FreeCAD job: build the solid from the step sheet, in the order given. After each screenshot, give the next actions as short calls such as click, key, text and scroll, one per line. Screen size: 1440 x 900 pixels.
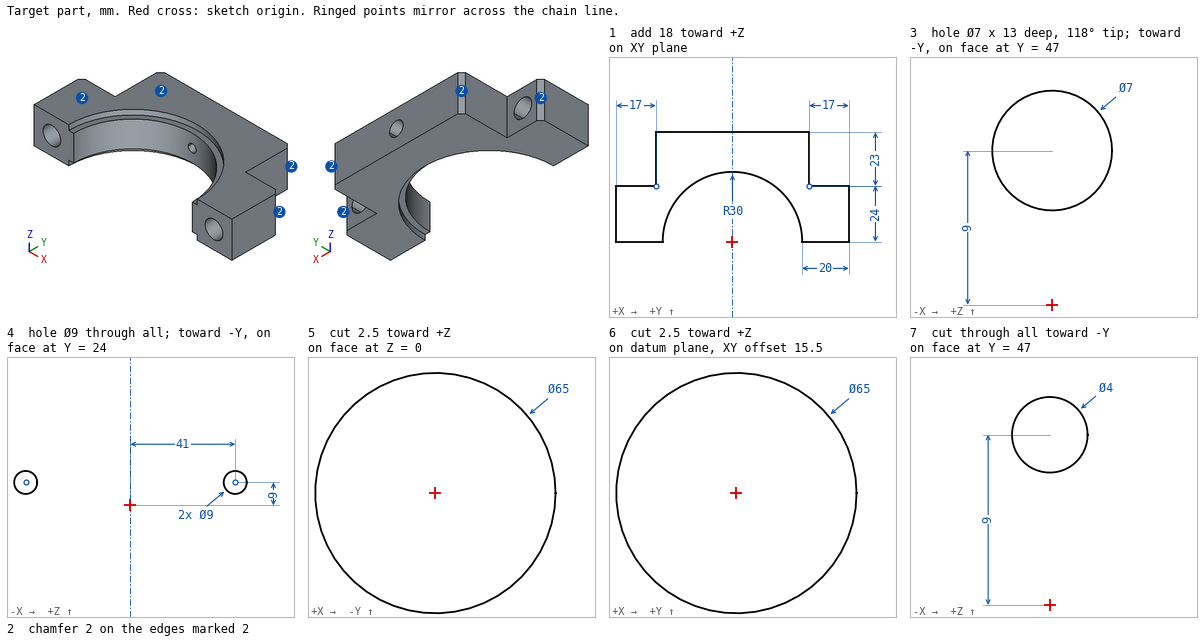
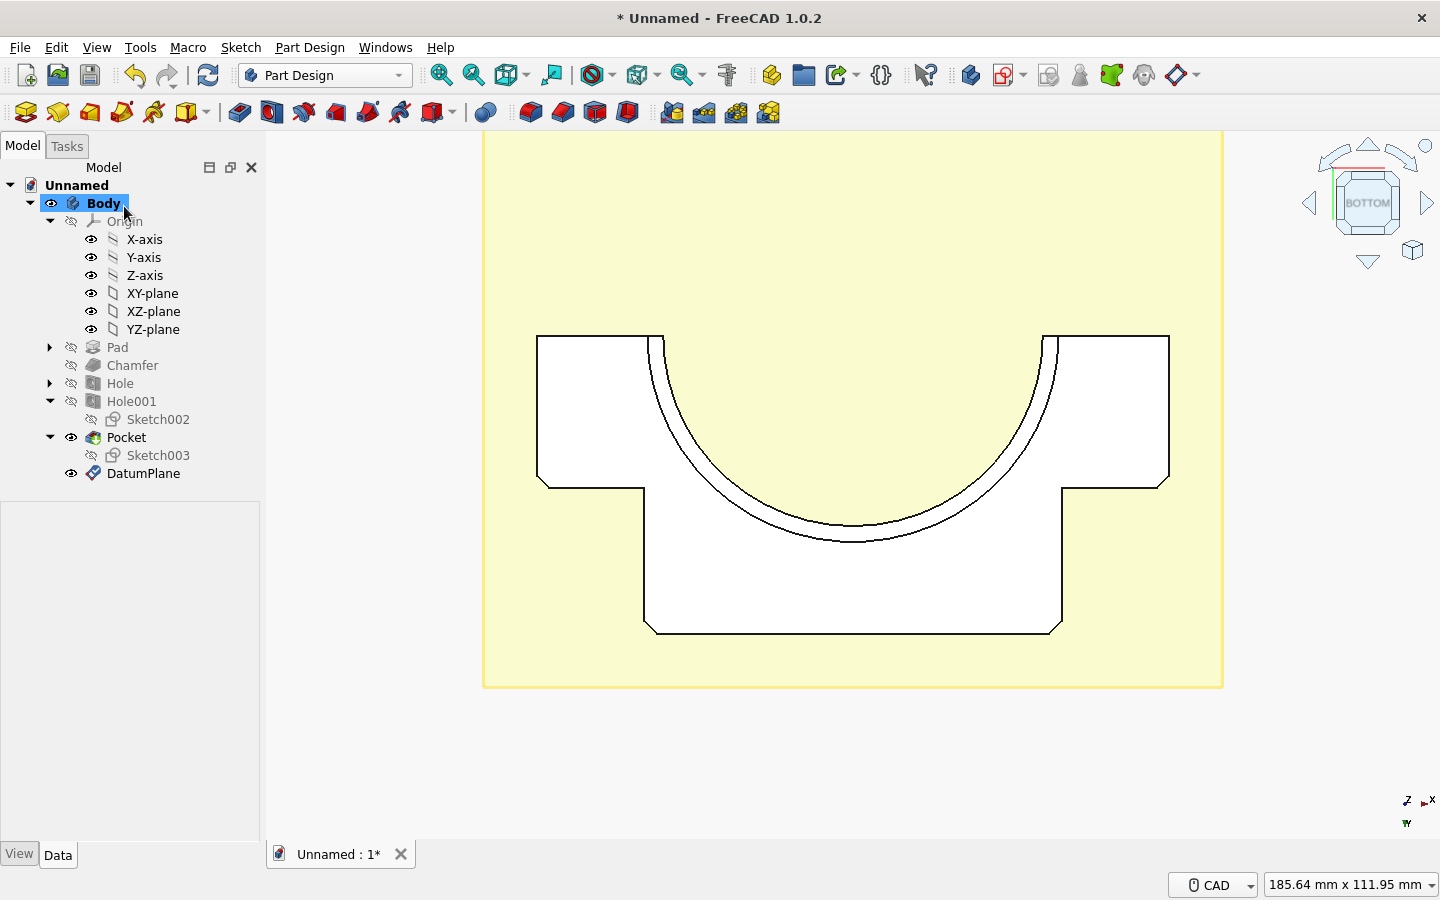
click(116, 473)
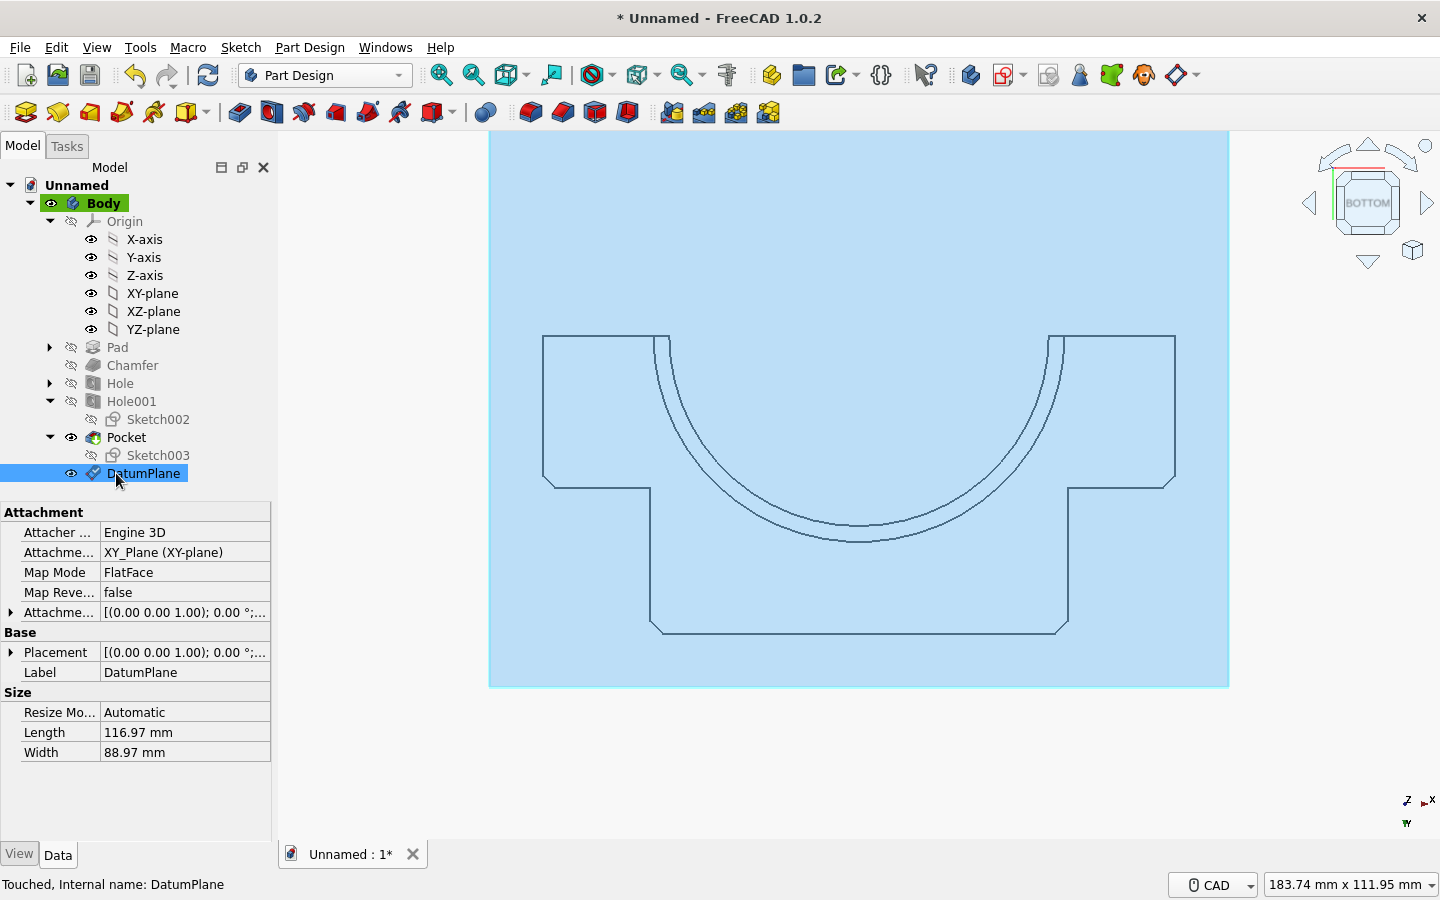
click(1004, 76)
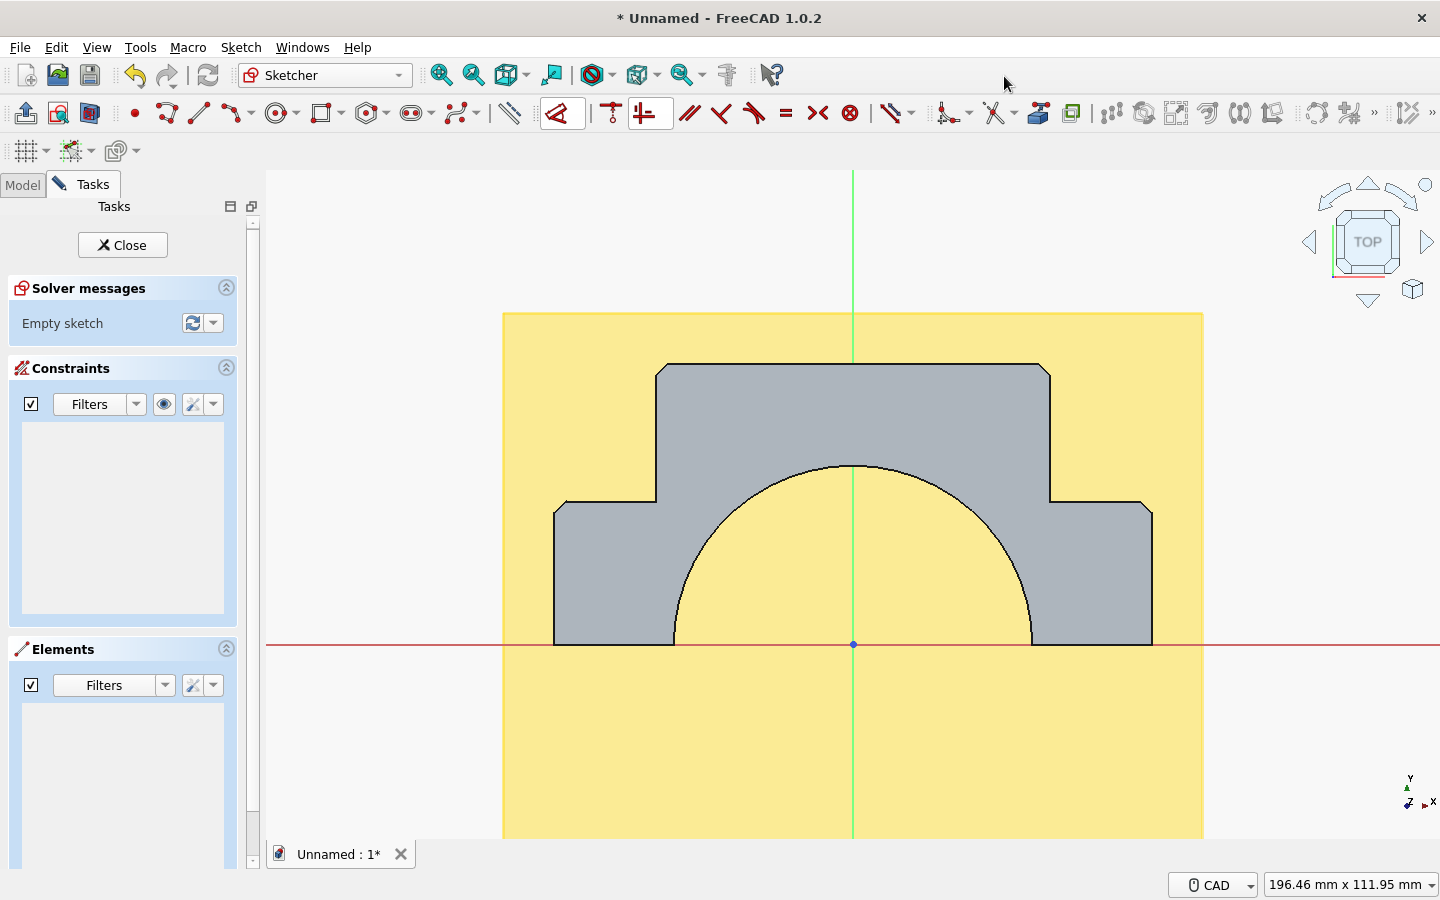
click(90, 114)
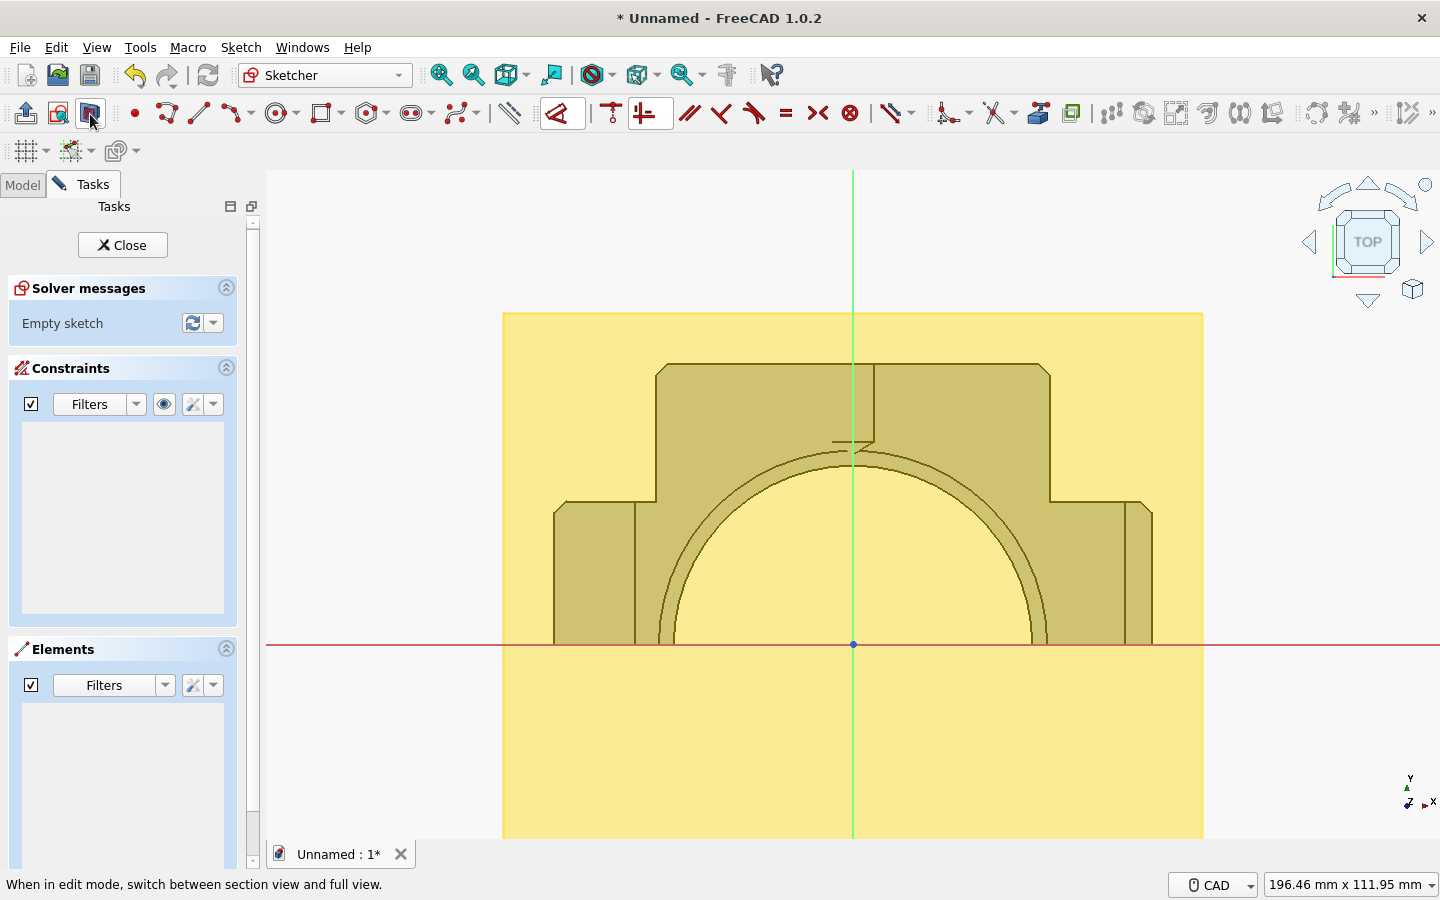
scroll(475, 198, down, 1)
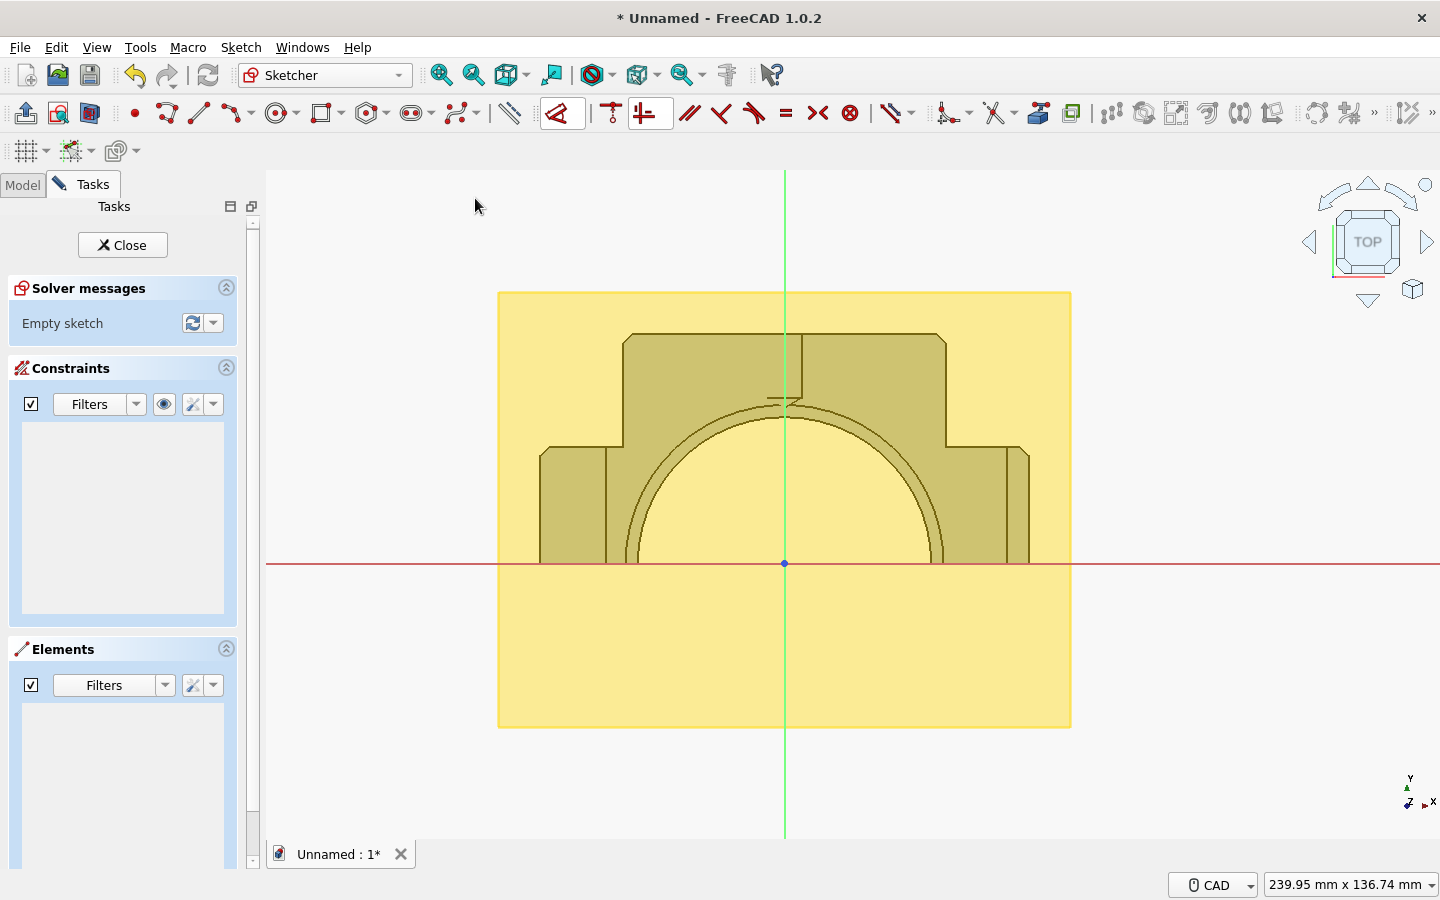
scroll(785, 685, up, 2)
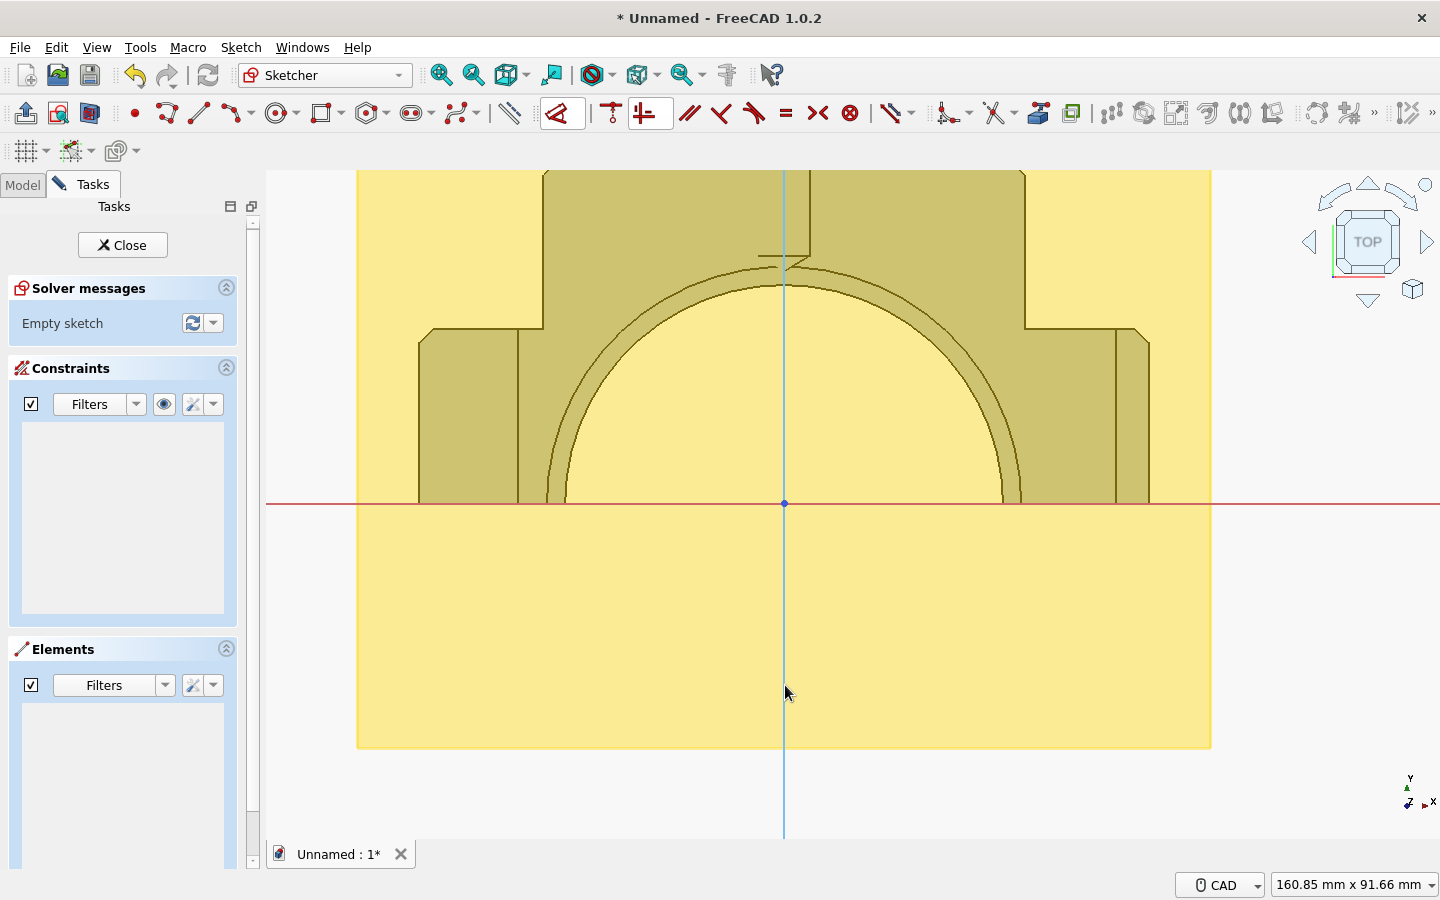
click(276, 114)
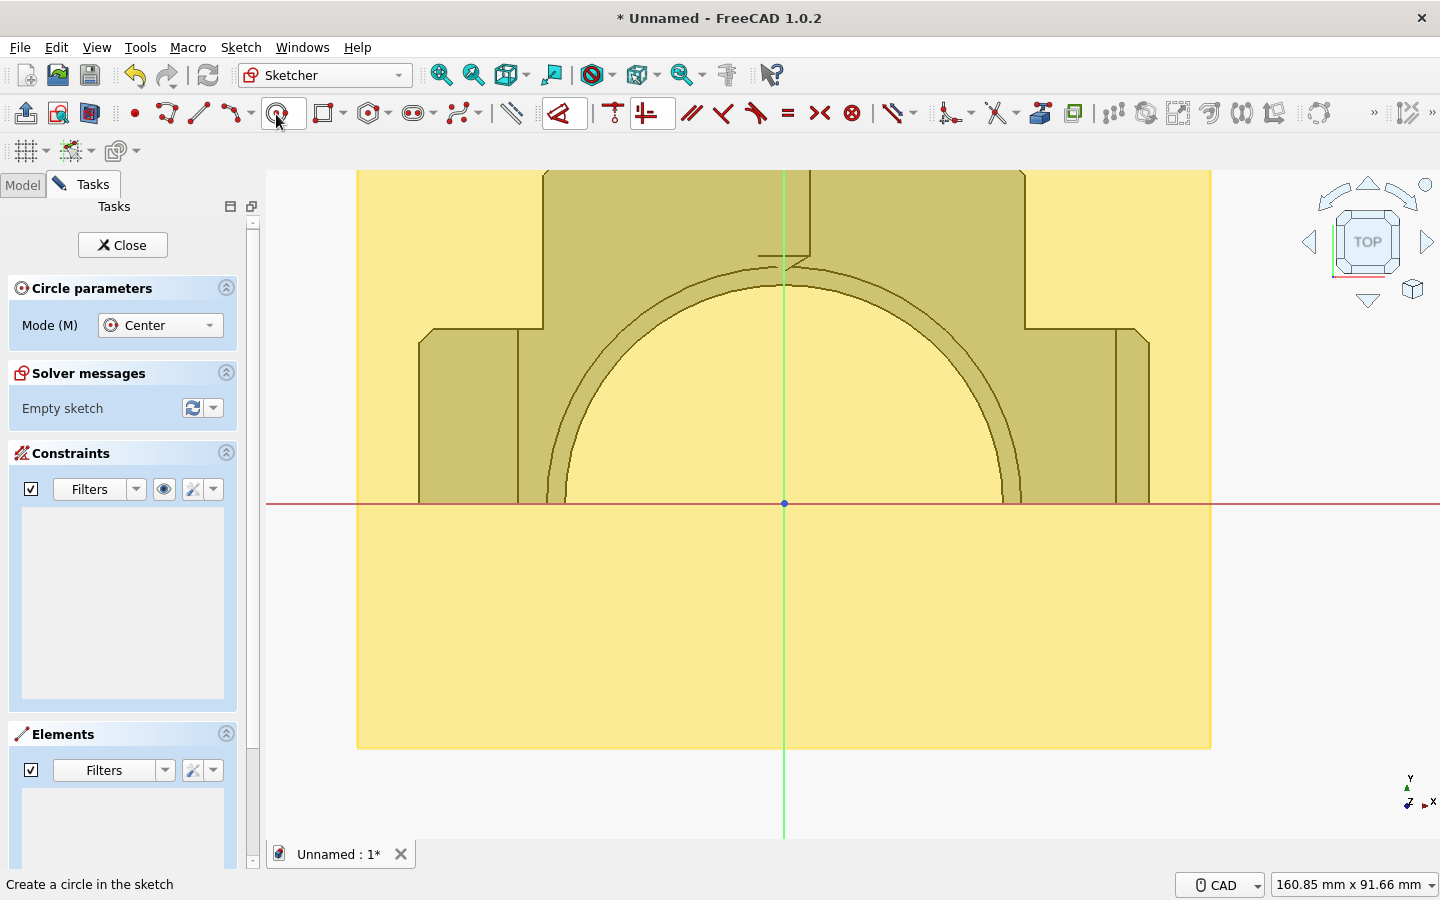
click(784, 504)
click(952, 336)
key(Escape)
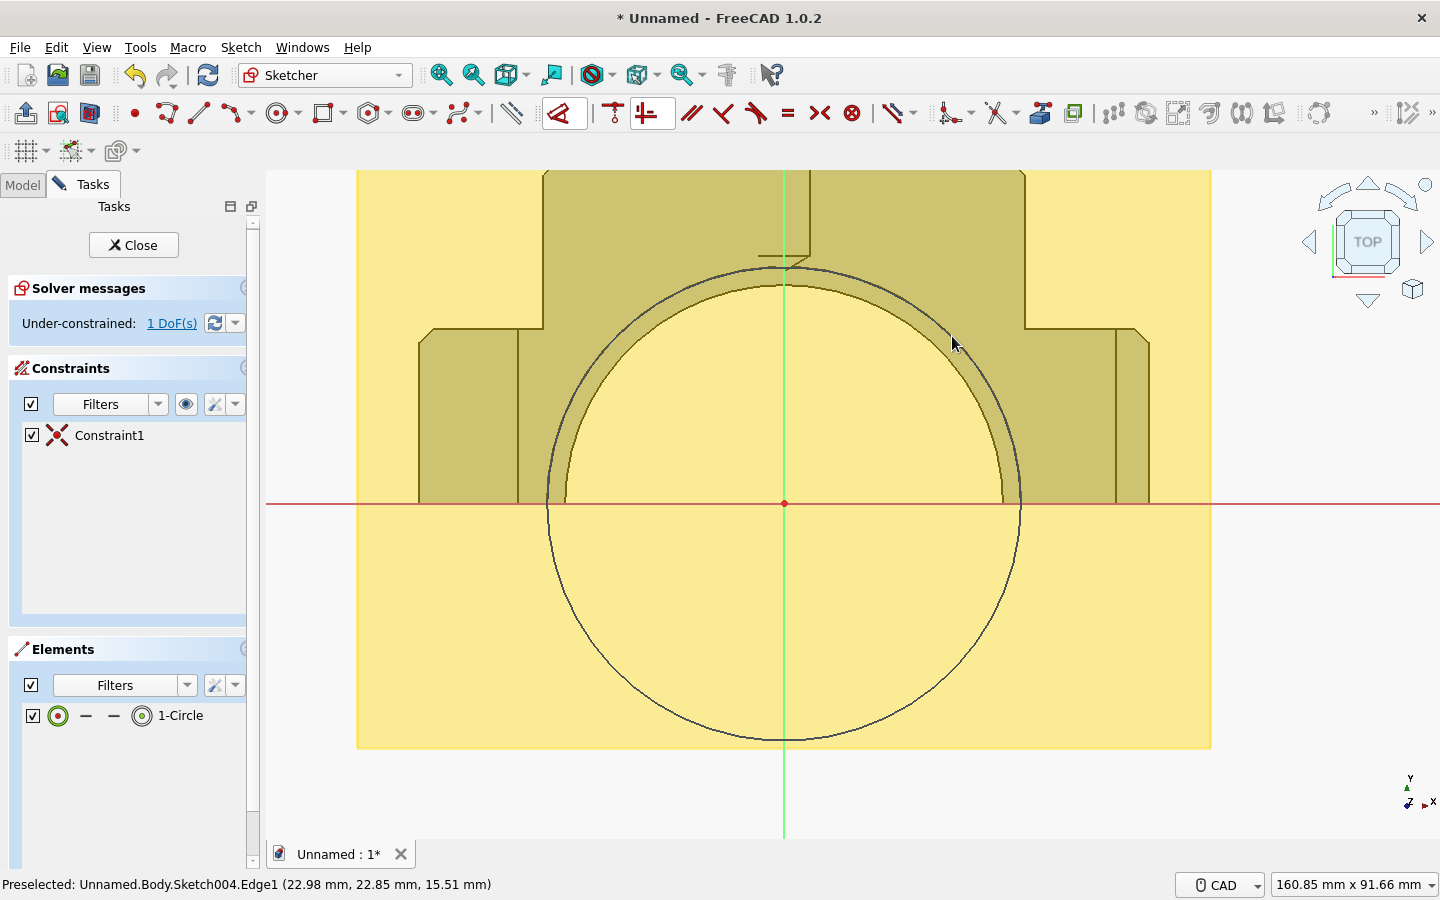
click(951, 336)